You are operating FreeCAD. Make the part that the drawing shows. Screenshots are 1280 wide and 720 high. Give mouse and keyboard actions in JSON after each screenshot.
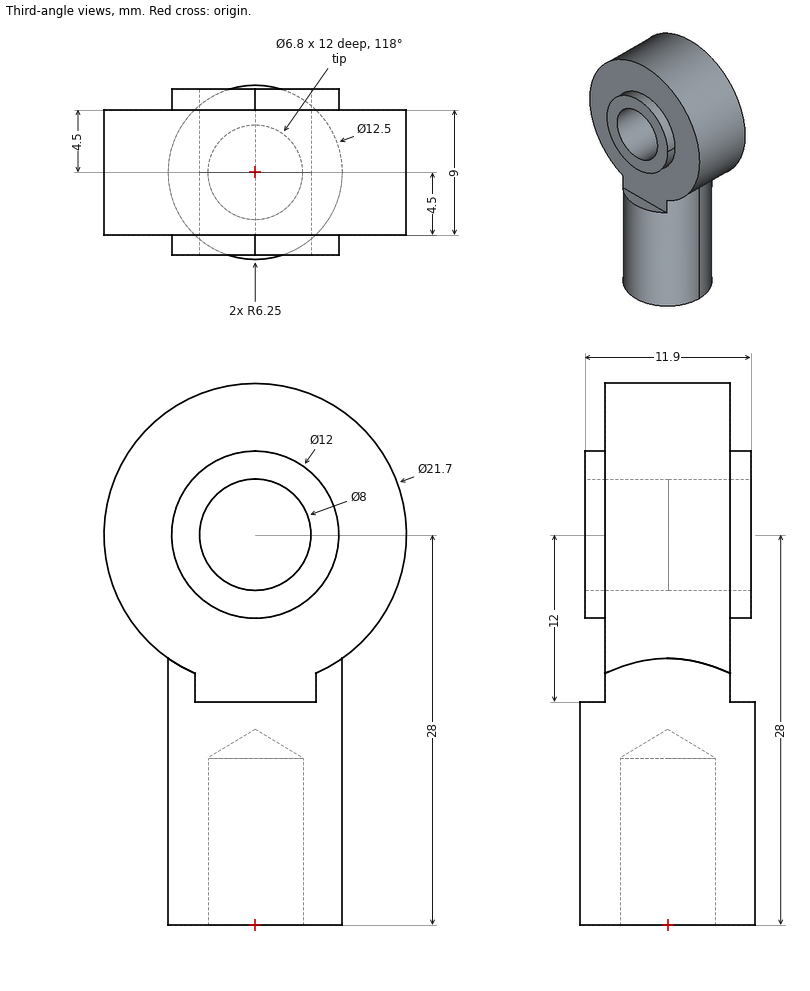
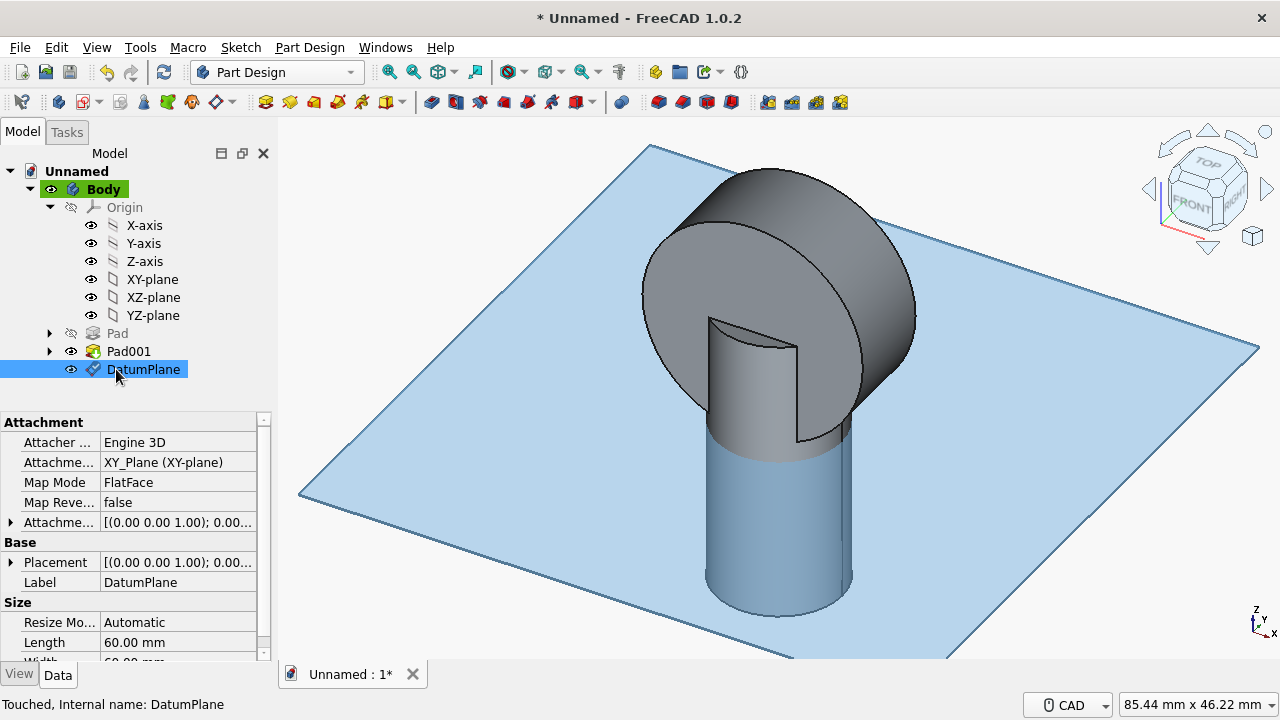
{"action": "left_click", "coordinate": [84, 102]}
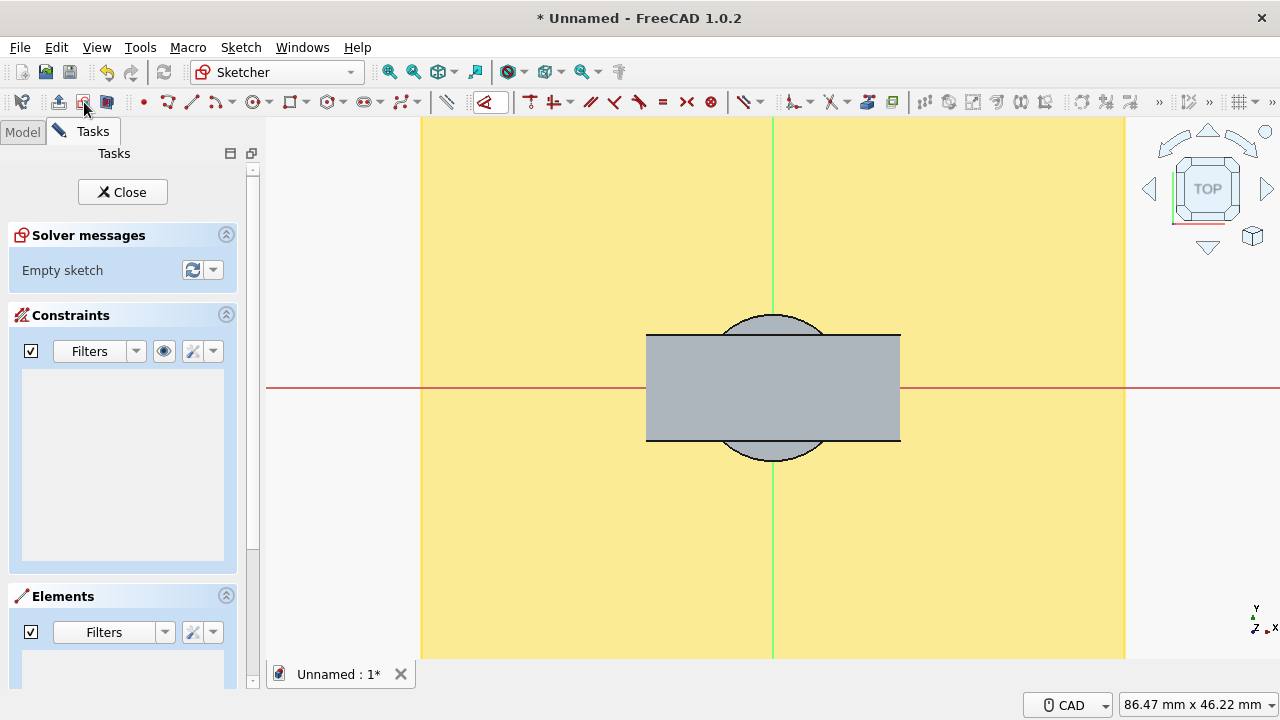
{"action": "key", "text": "q s"}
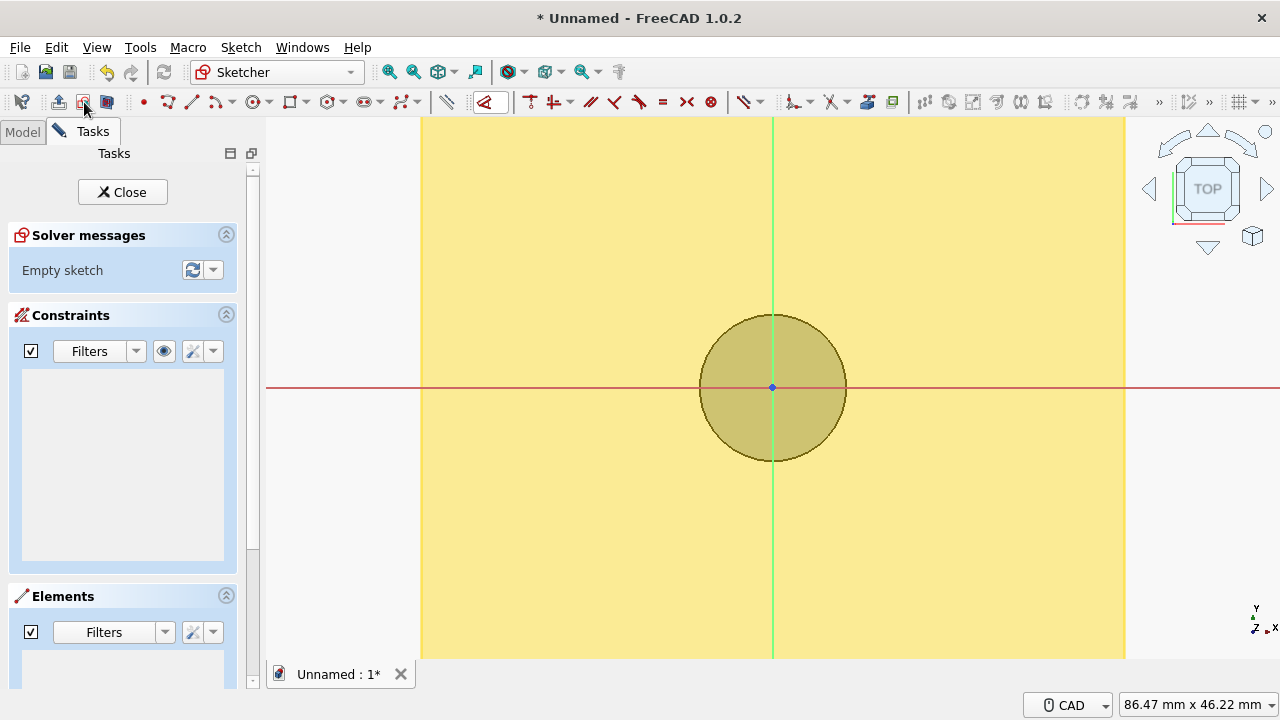
{"action": "scroll", "coordinate": [829, 388], "scroll_direction": "up", "scroll_amount": 4}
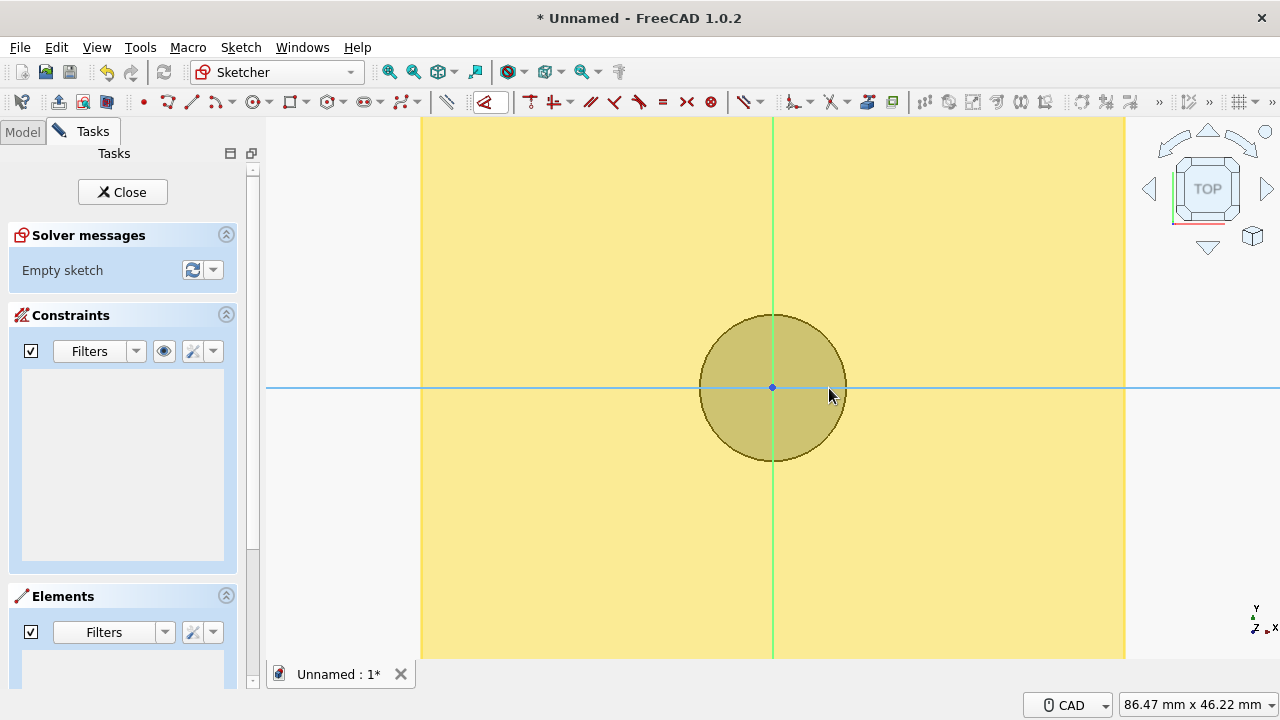
{"action": "key", "text": "g l"}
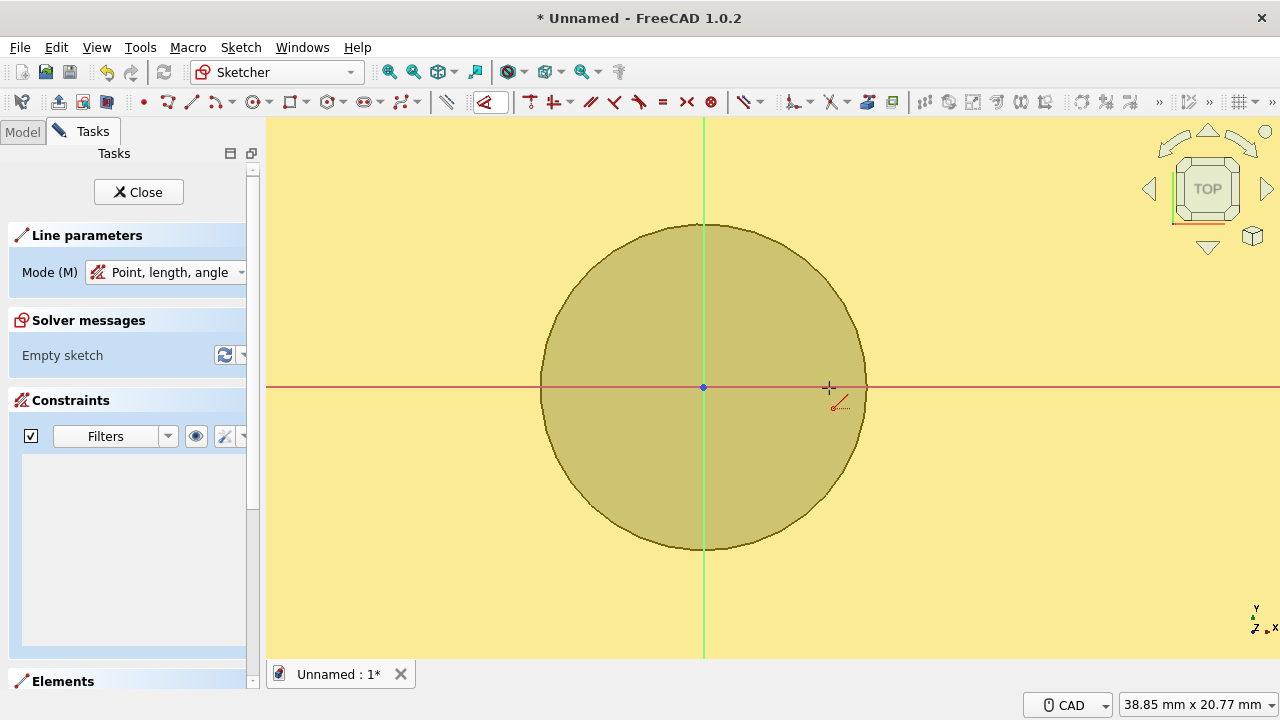
{"action": "left_click", "coordinate": [817, 505]}
{"action": "left_click", "coordinate": [590, 505]}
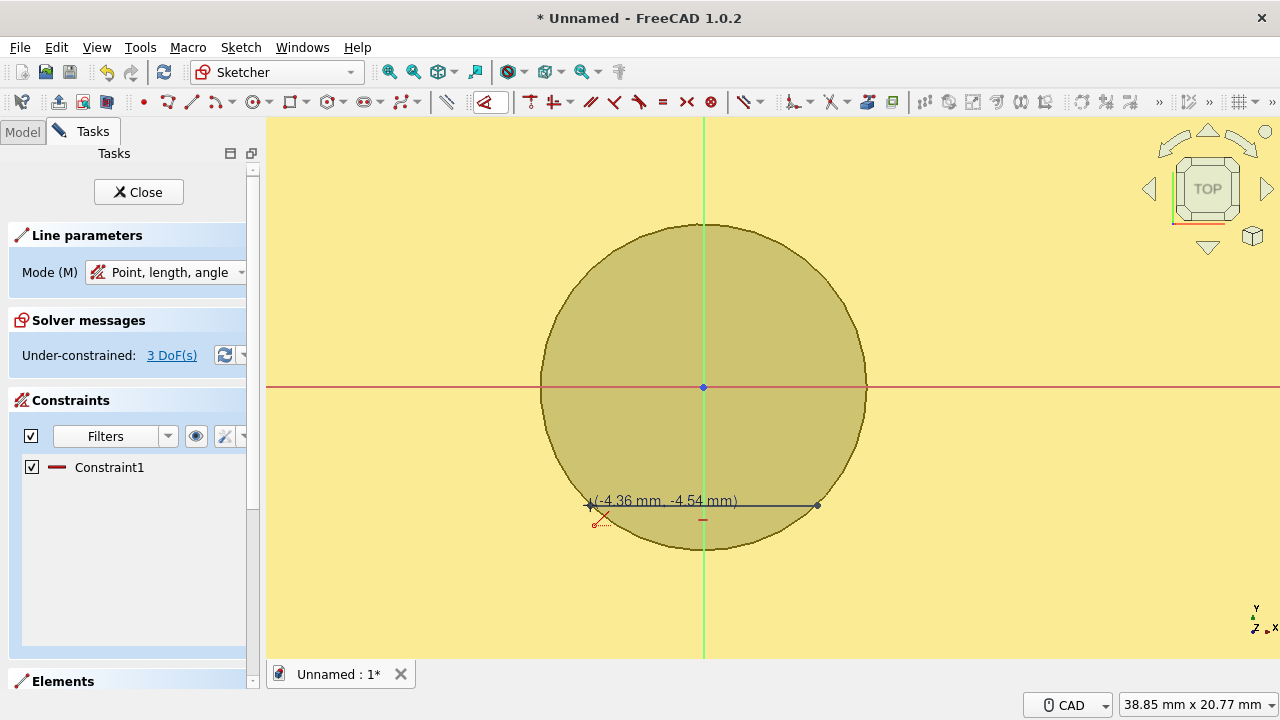
{"action": "key", "text": "g 3 a"}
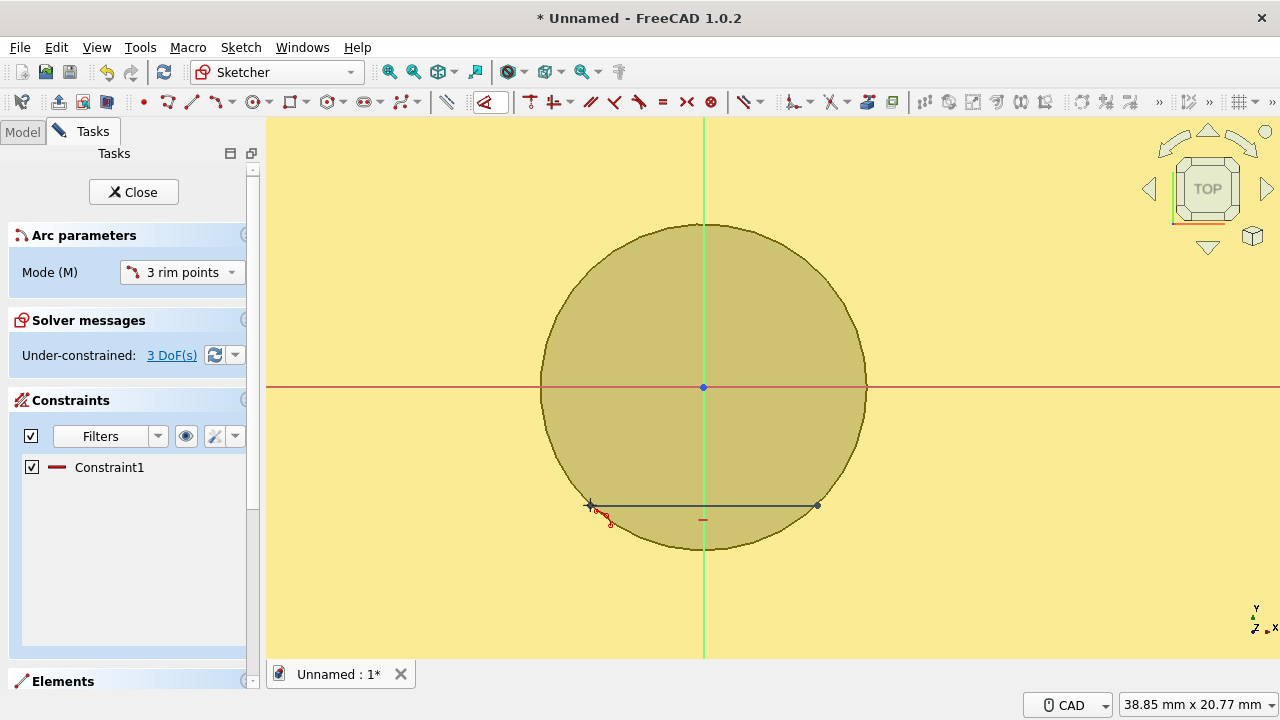
{"action": "left_click", "coordinate": [590, 506]}
{"action": "left_click", "coordinate": [817, 506]}
{"action": "left_click", "coordinate": [679, 549]}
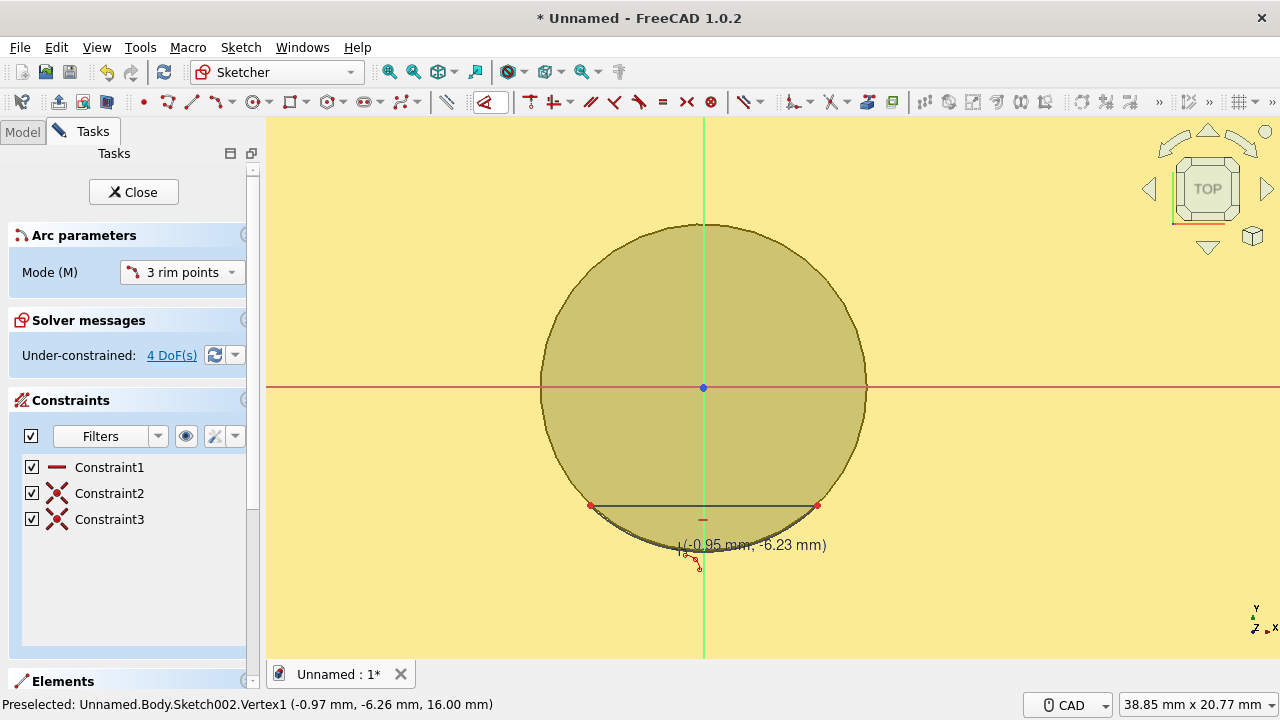
{"action": "key", "text": "g l"}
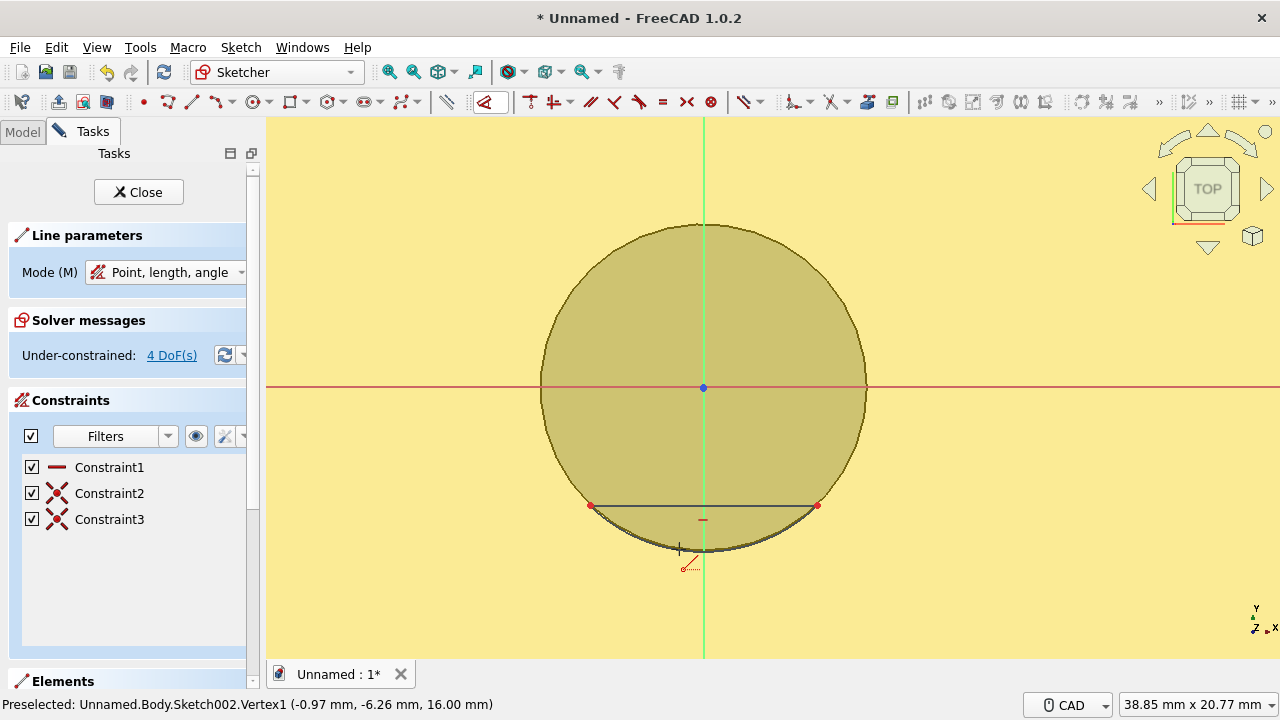
{"action": "left_click", "coordinate": [590, 270]}
{"action": "left_click", "coordinate": [817, 270]}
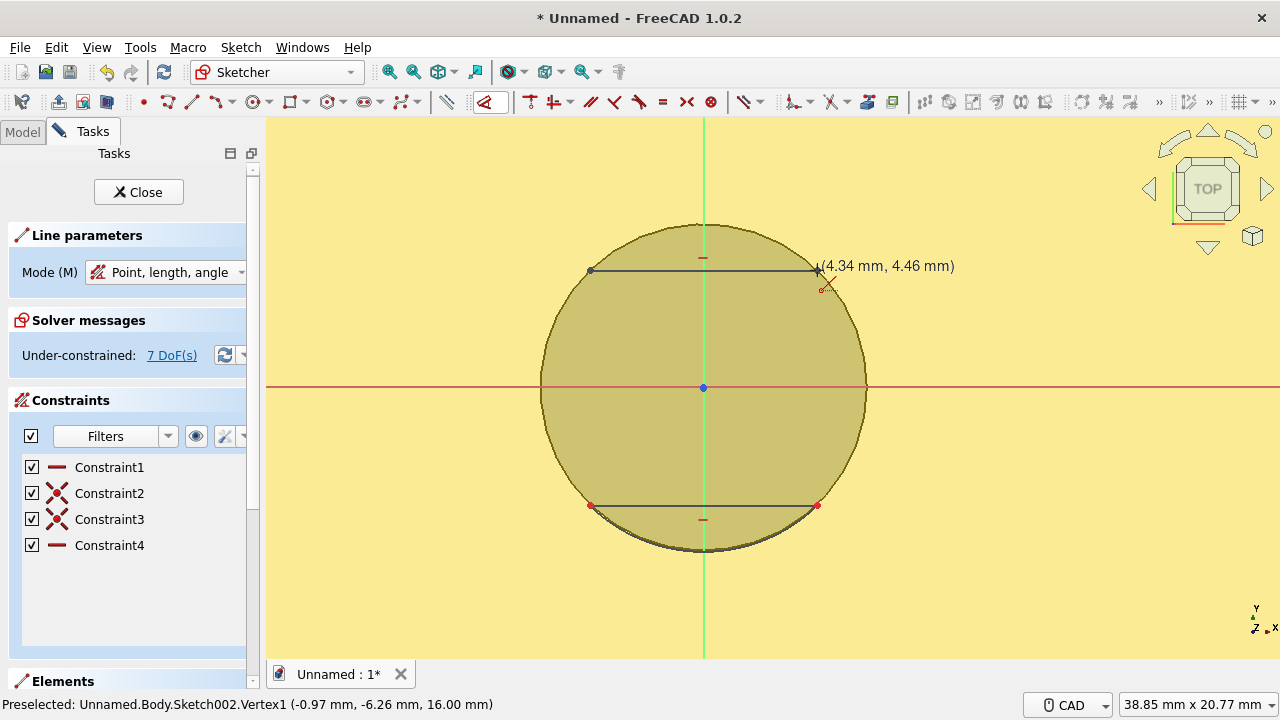
{"action": "key", "text": "g 3 a"}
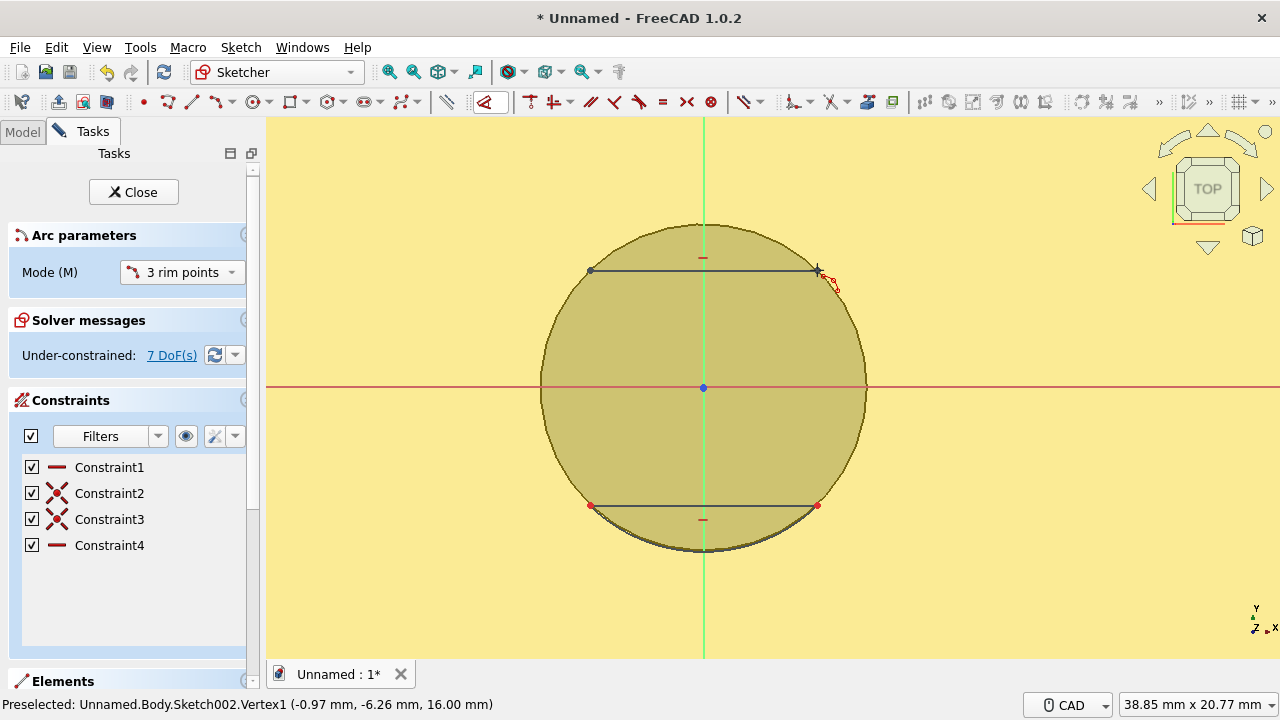
{"action": "left_click", "coordinate": [817, 271]}
{"action": "left_click", "coordinate": [590, 271]}
{"action": "left_click", "coordinate": [729, 226]}
{"action": "key", "text": "Escape"}